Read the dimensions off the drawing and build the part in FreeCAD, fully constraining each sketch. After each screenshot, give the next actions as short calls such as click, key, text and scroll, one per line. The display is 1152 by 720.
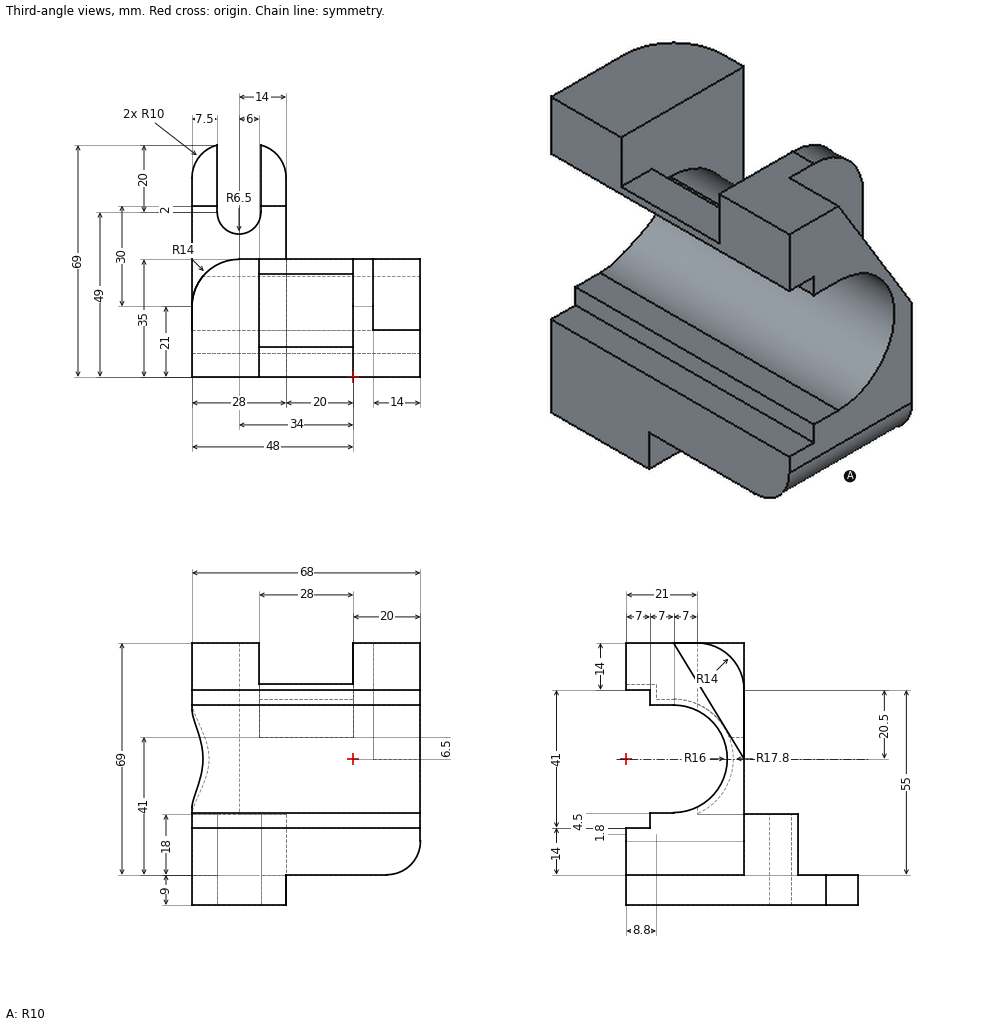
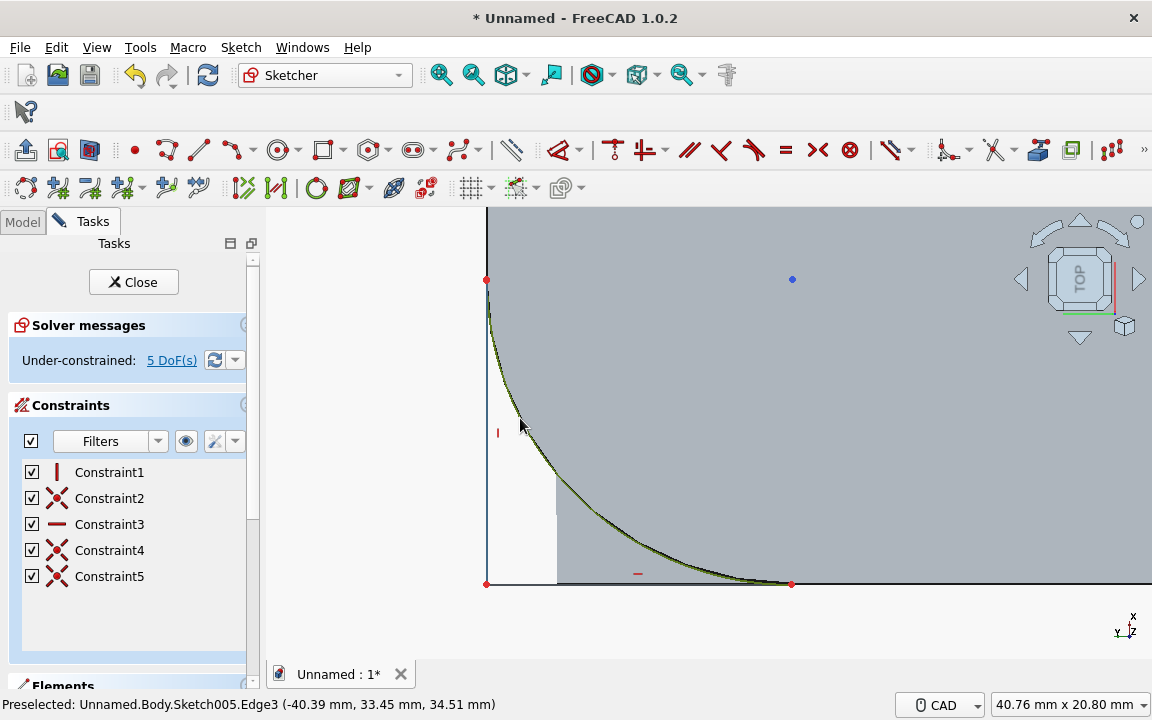
click(754, 150)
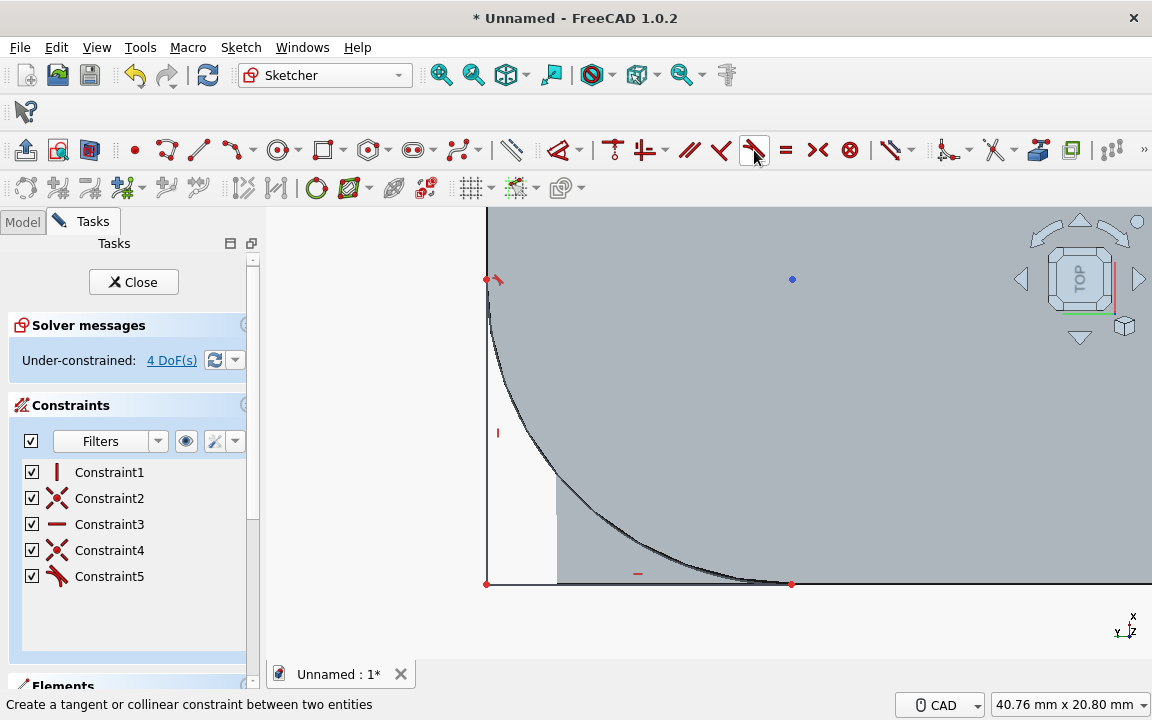
click(578, 585)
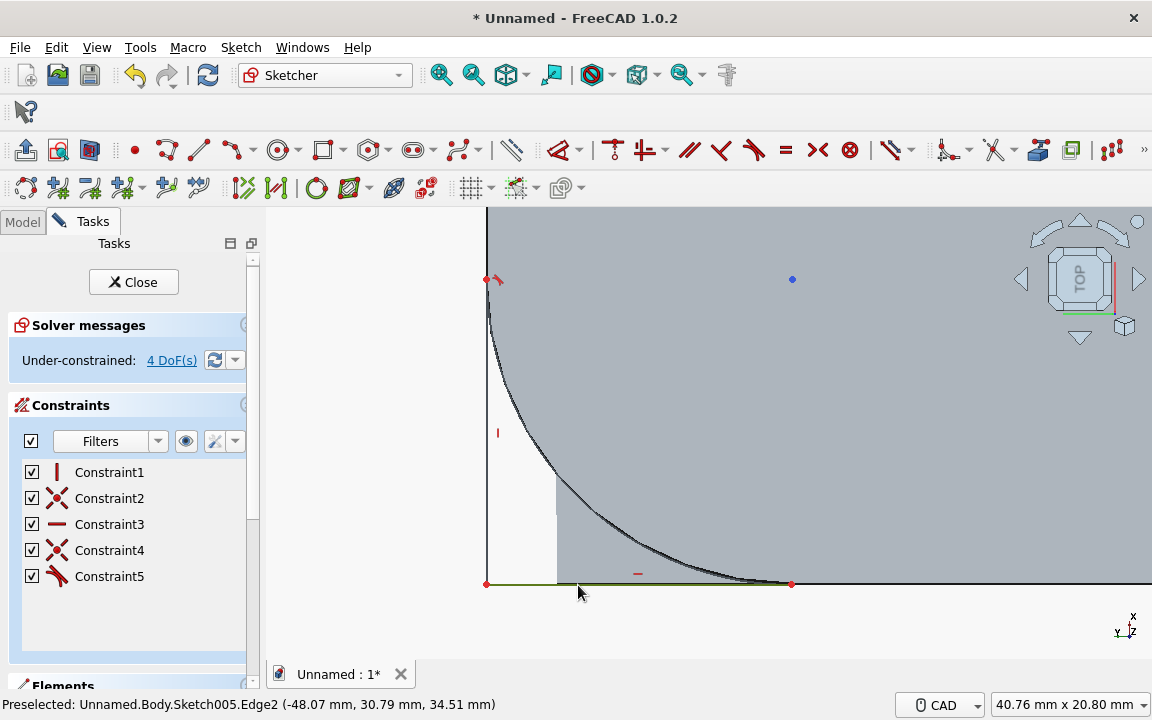
click(520, 418)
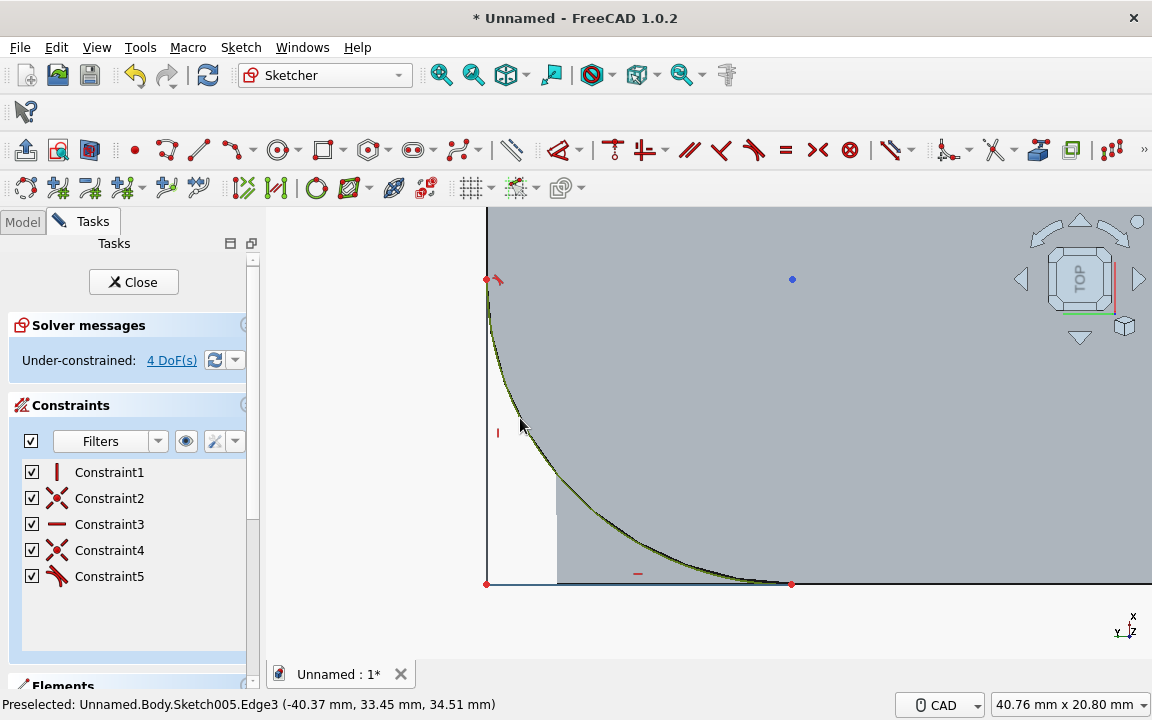
click(754, 150)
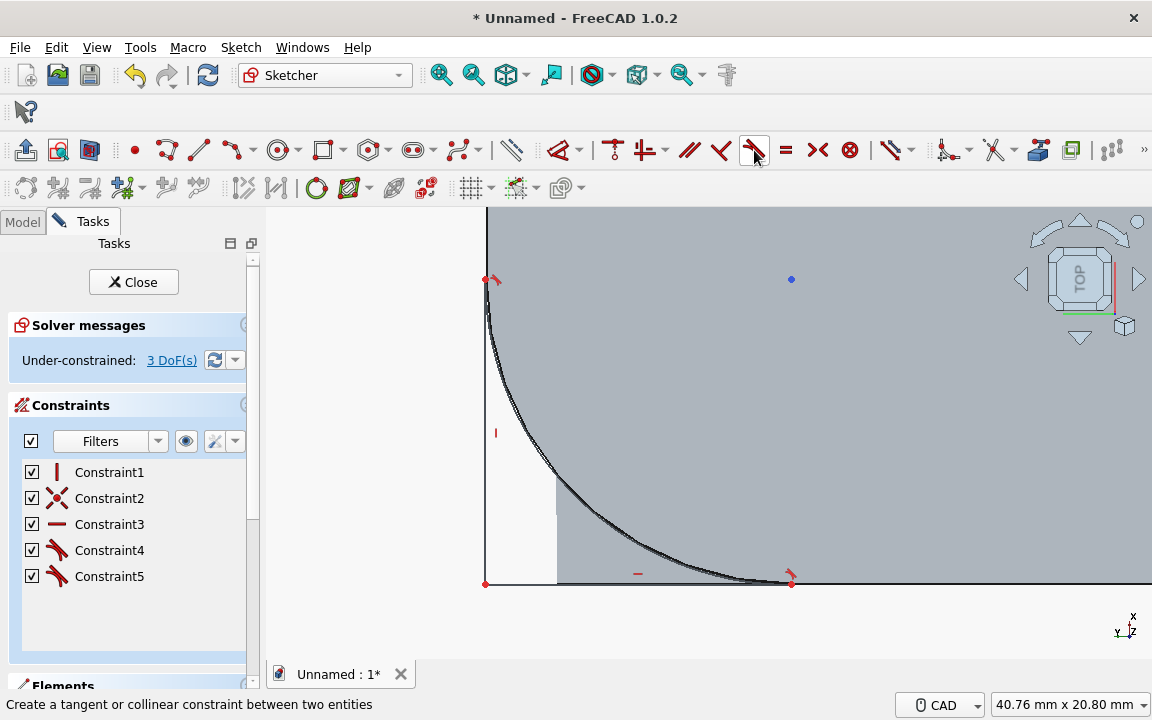
key(d)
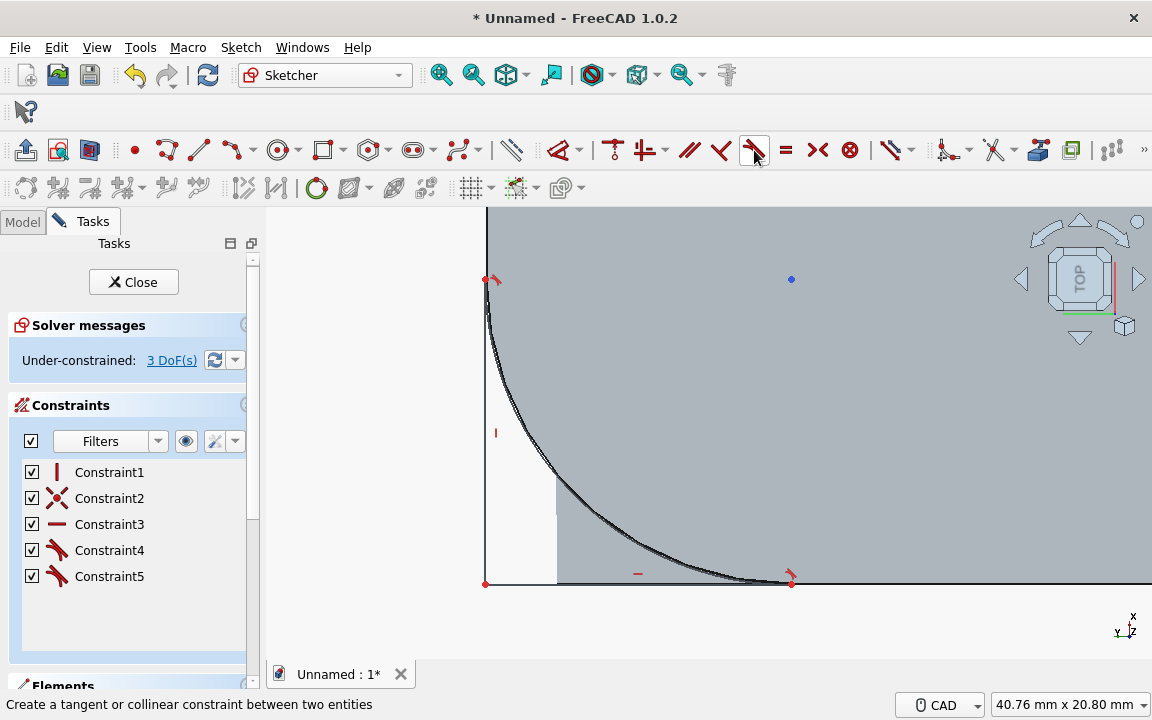
click(519, 418)
click(454, 270)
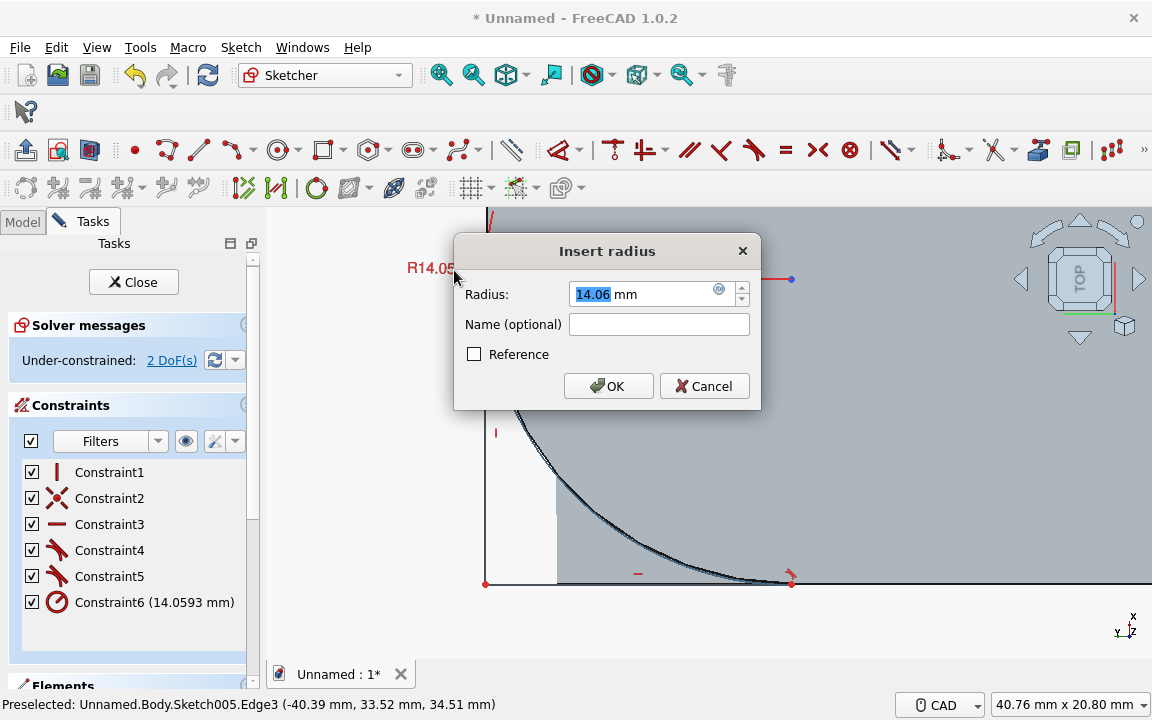
text(14)
key(Return)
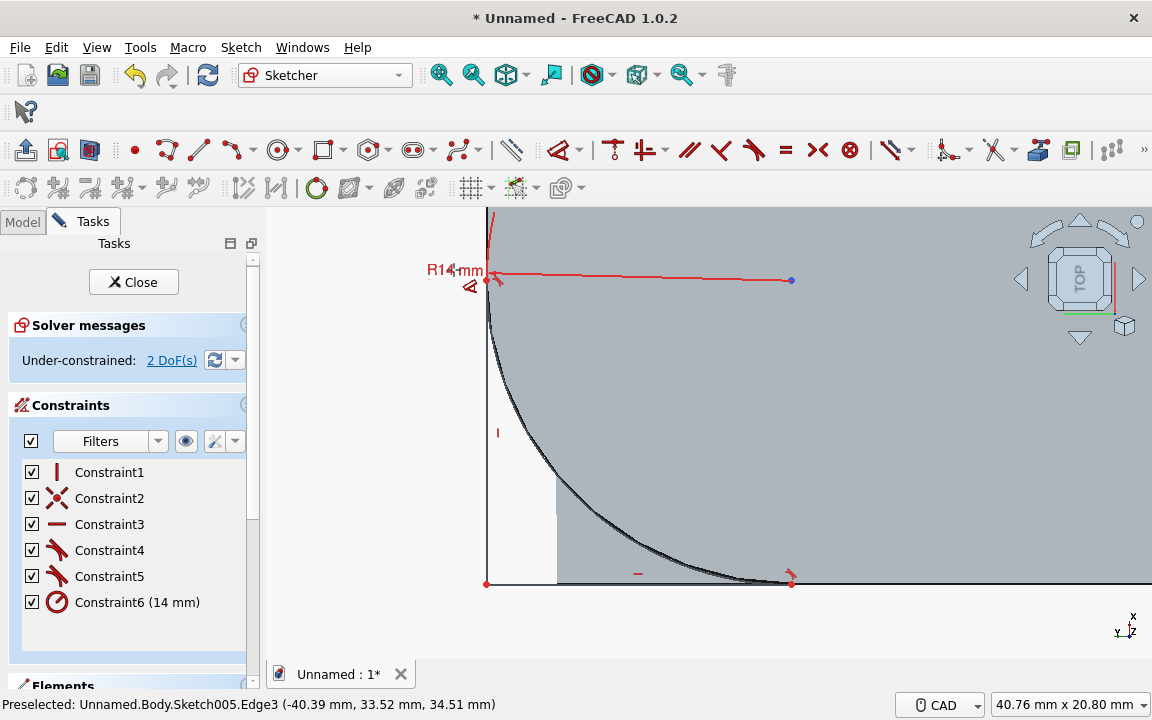
click(487, 281)
click(737, 315)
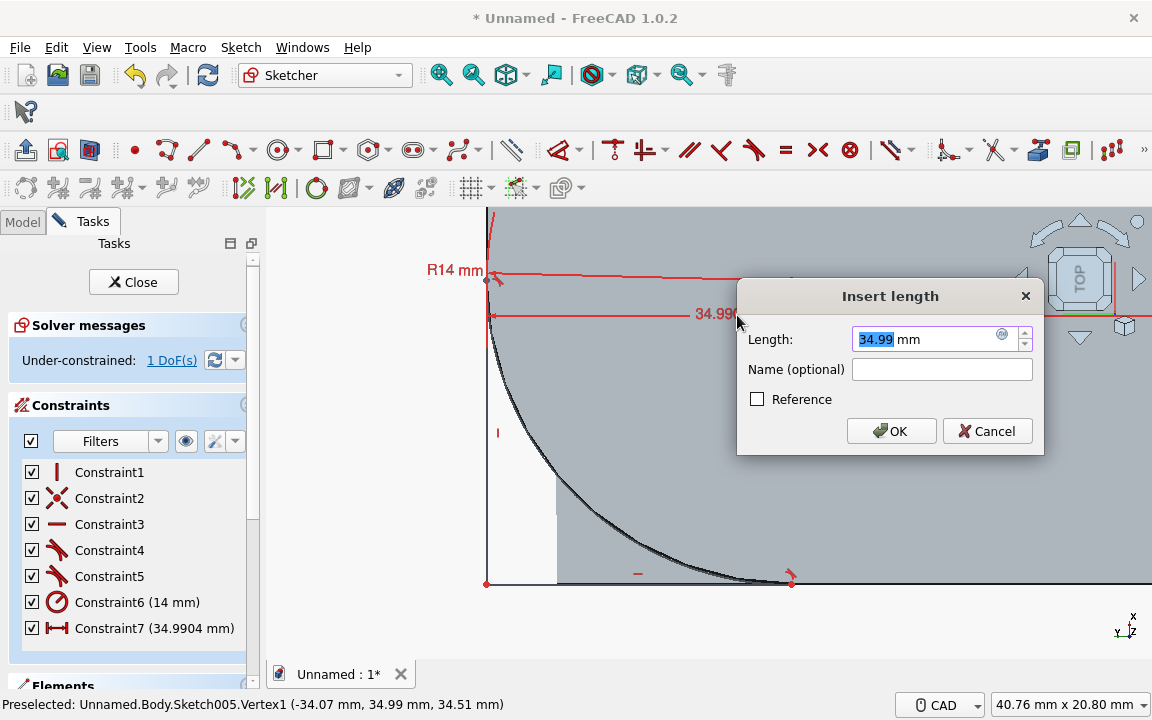
text(35)
key(Return)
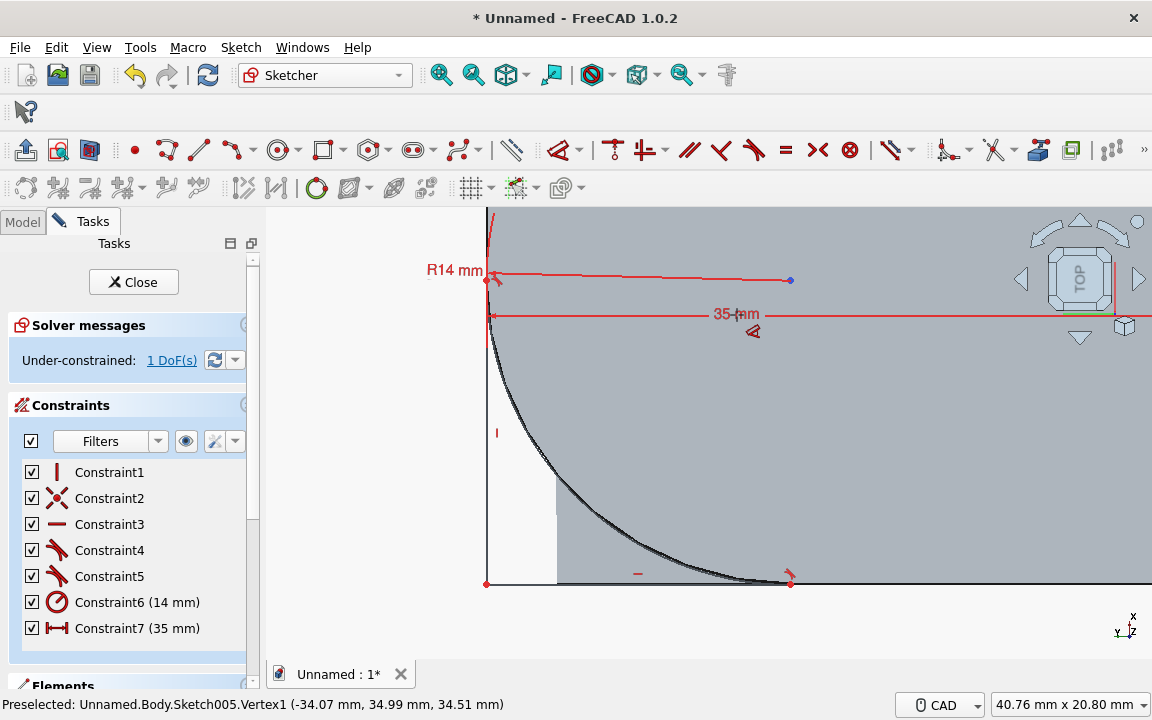
click(487, 281)
click(453, 247)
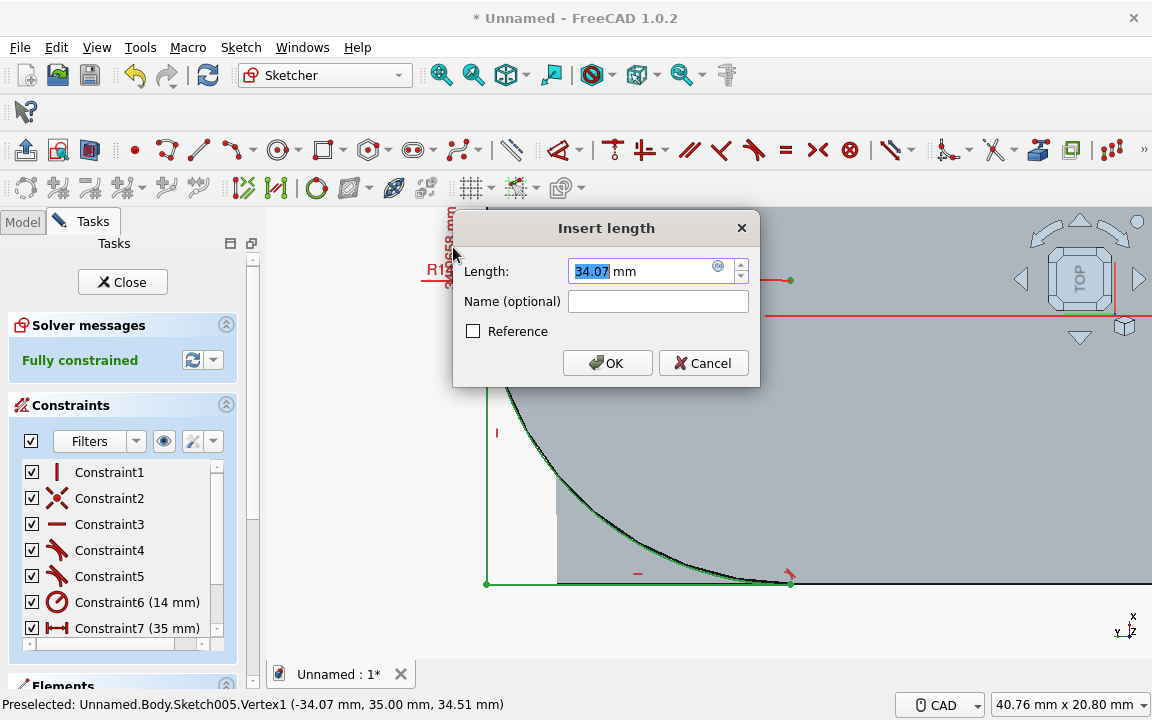
text(34)
key(Return)
key(Escape)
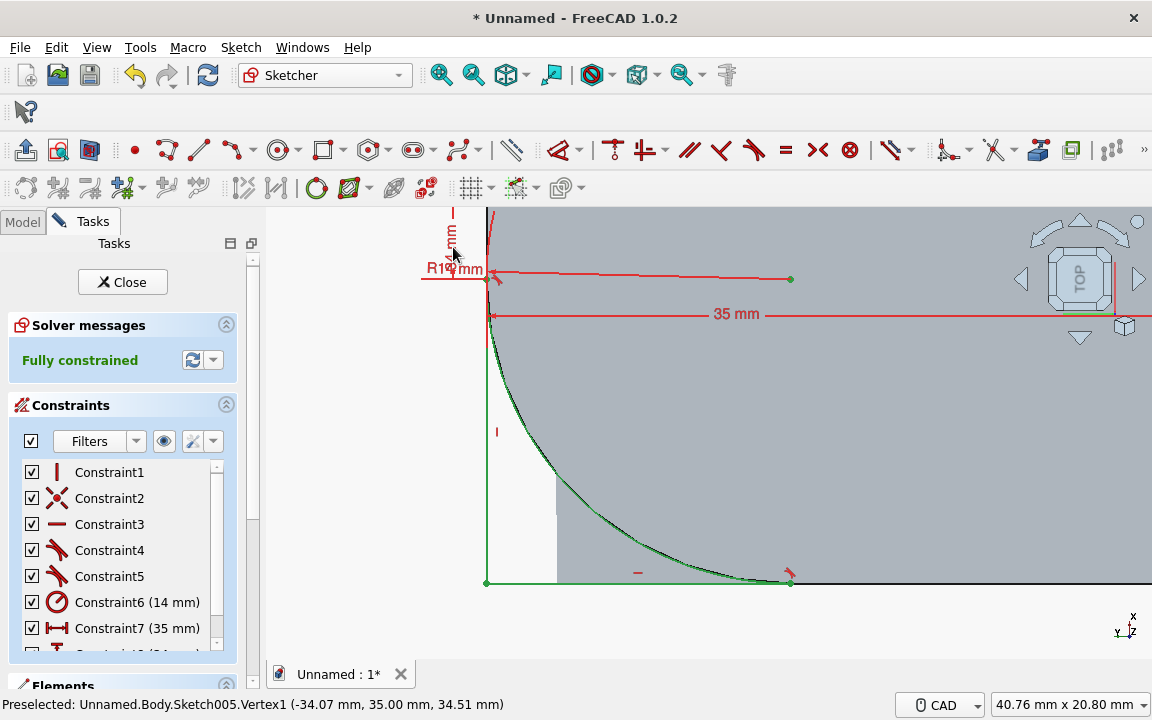
click(123, 282)